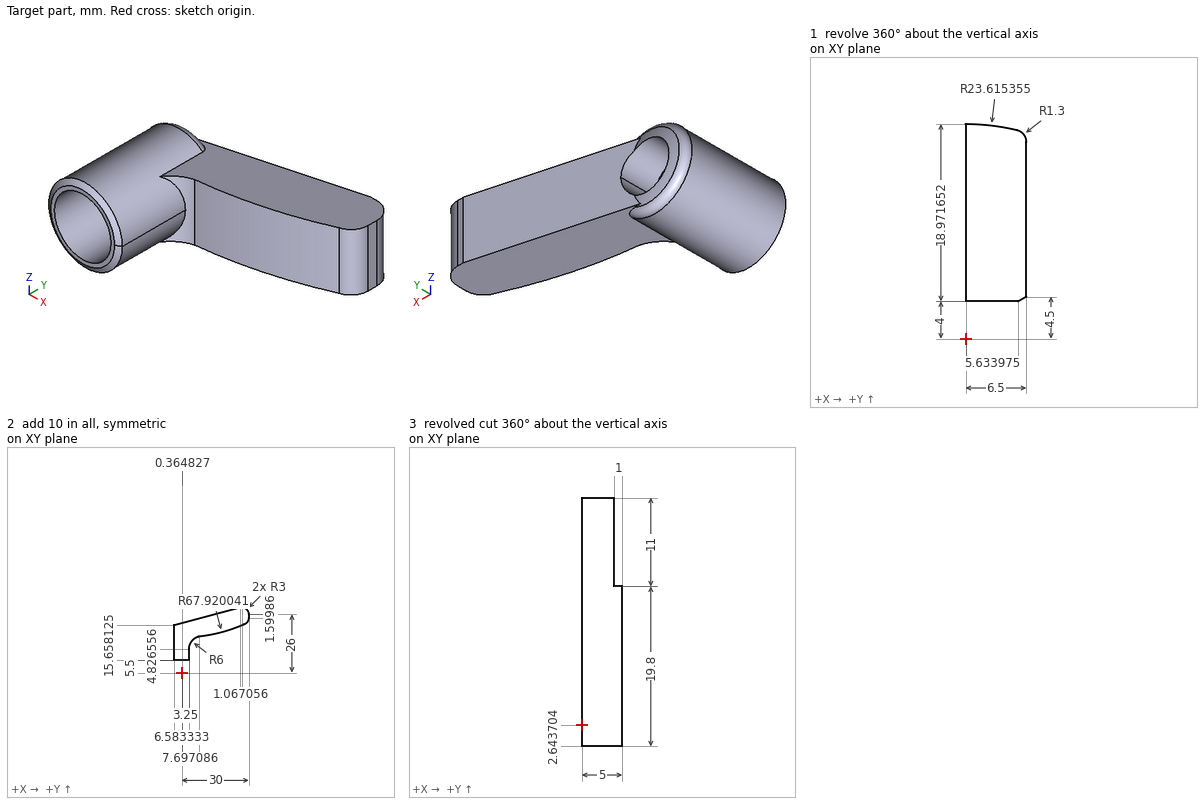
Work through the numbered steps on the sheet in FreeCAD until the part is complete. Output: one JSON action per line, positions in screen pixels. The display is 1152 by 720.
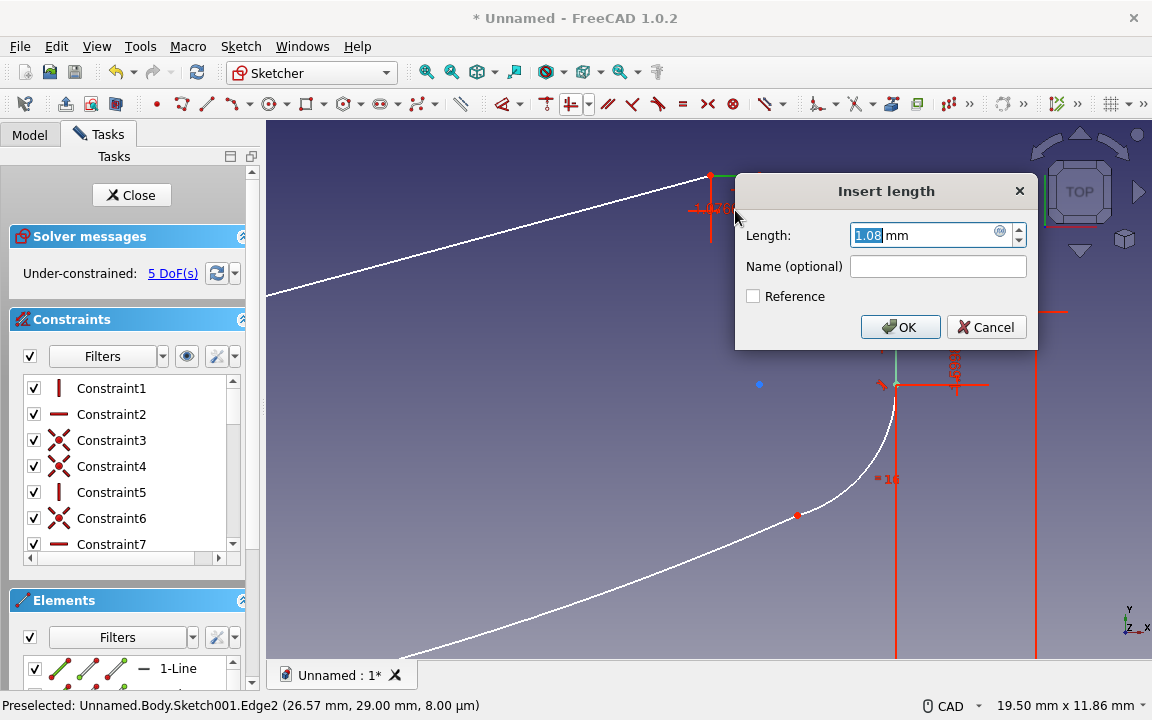
{"action": "type", "text": "1.067056"}
{"action": "key", "text": "Return"}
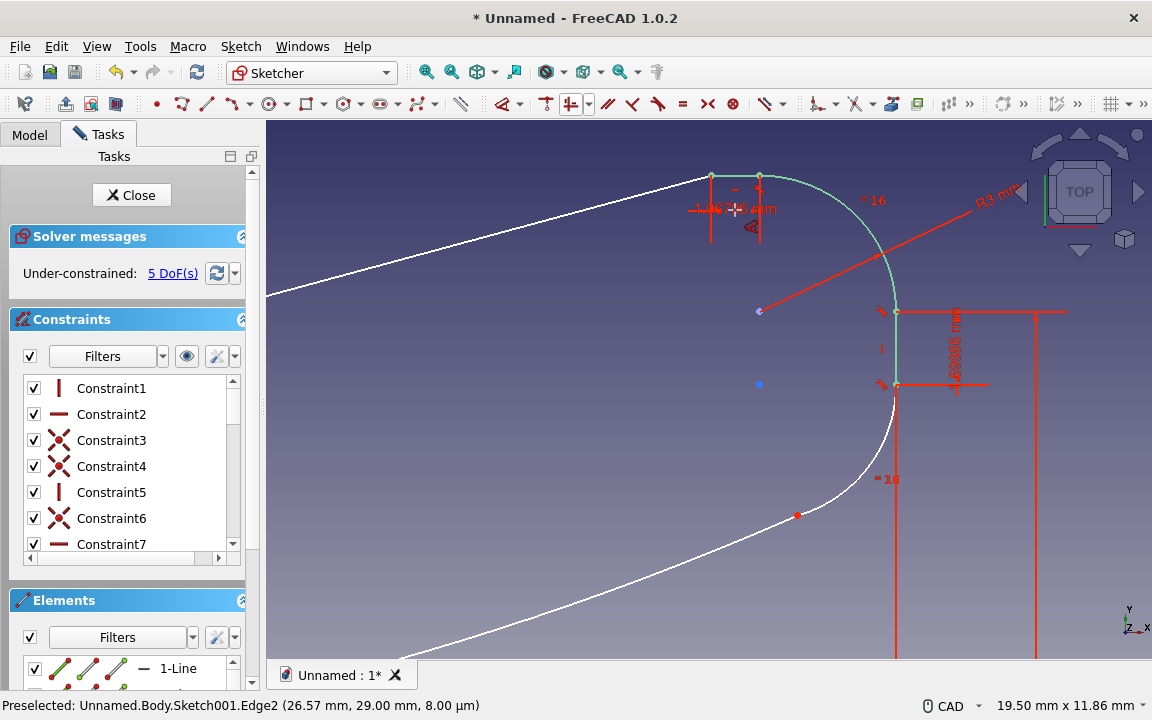
{"action": "scroll", "coordinate": [805, 244], "scroll_direction": "down", "scroll_amount": 7}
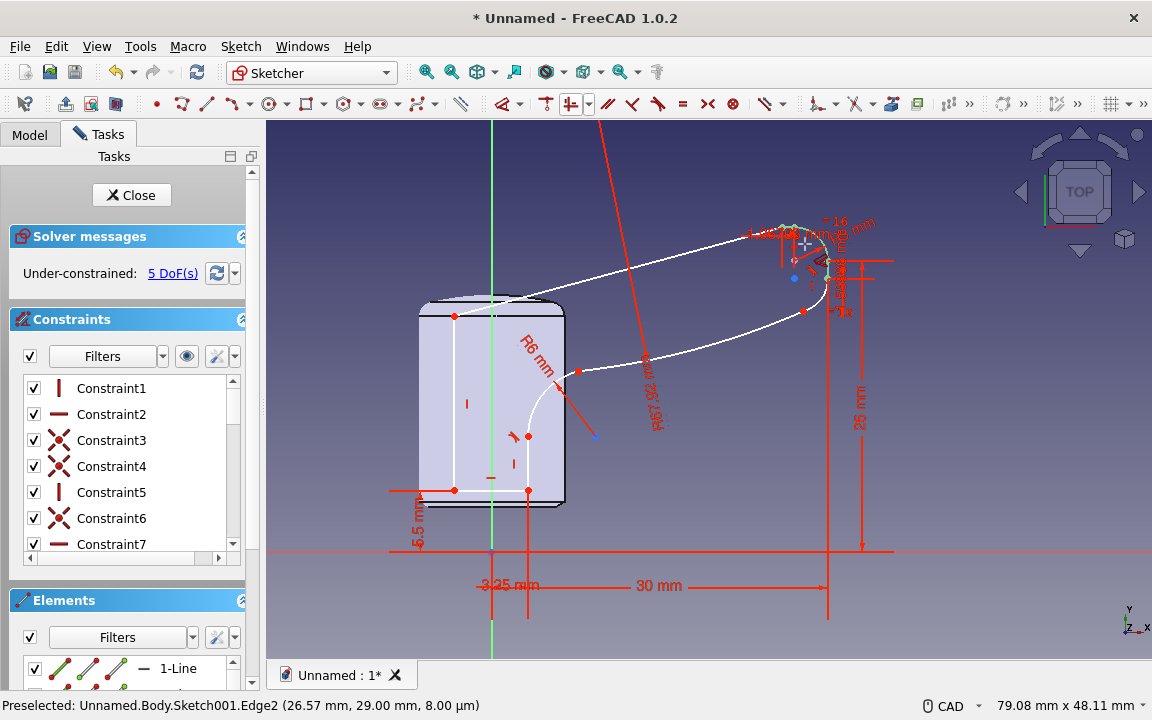
{"action": "left_click", "coordinate": [477, 491]}
{"action": "left_click", "coordinate": [508, 525]}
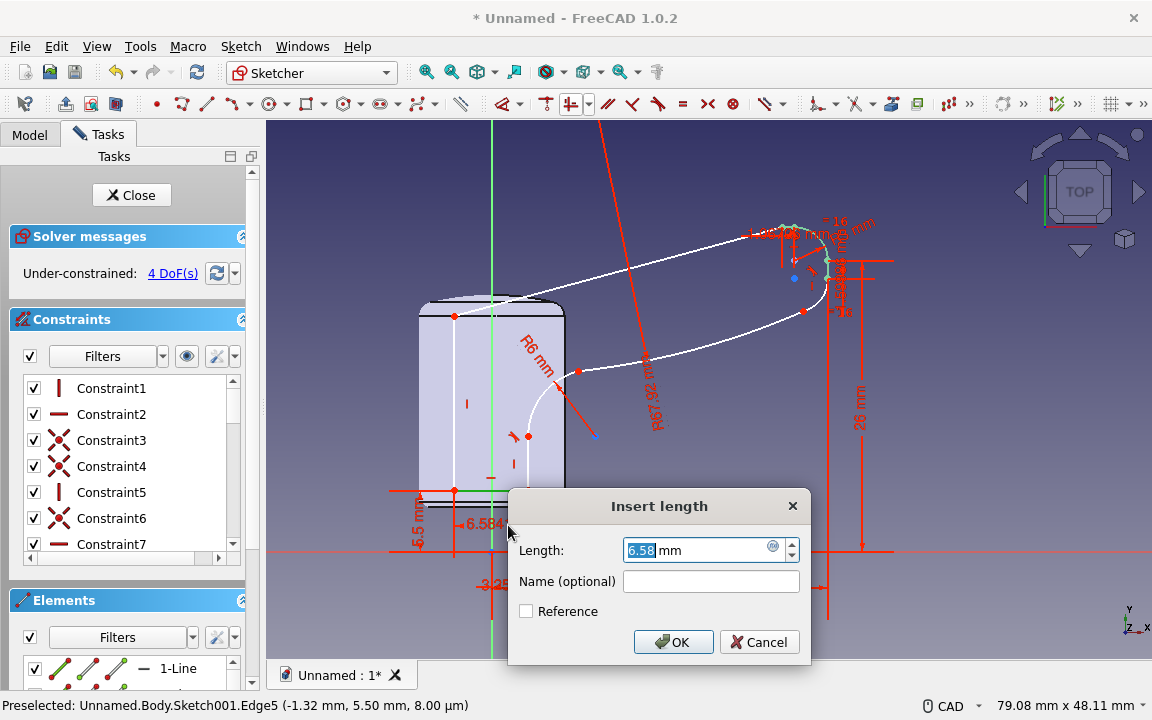
{"action": "type", "text": "6.583333"}
{"action": "key", "text": "Return"}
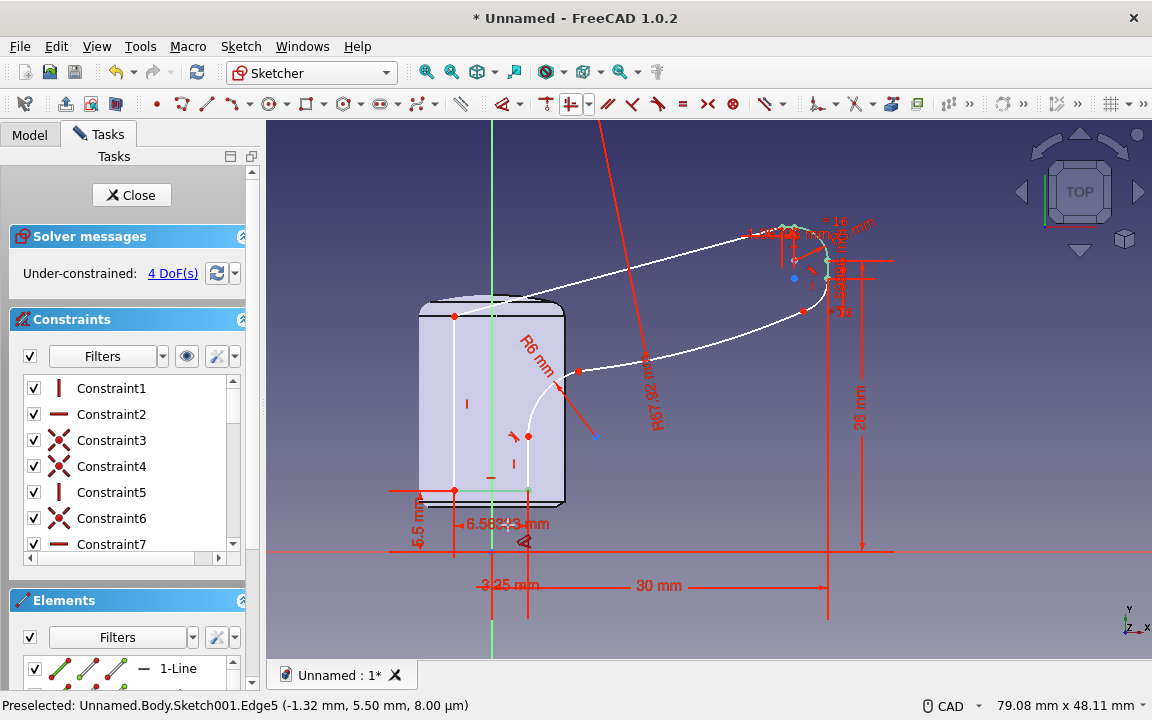
{"action": "left_click", "coordinate": [528, 474]}
{"action": "left_click", "coordinate": [562, 463]}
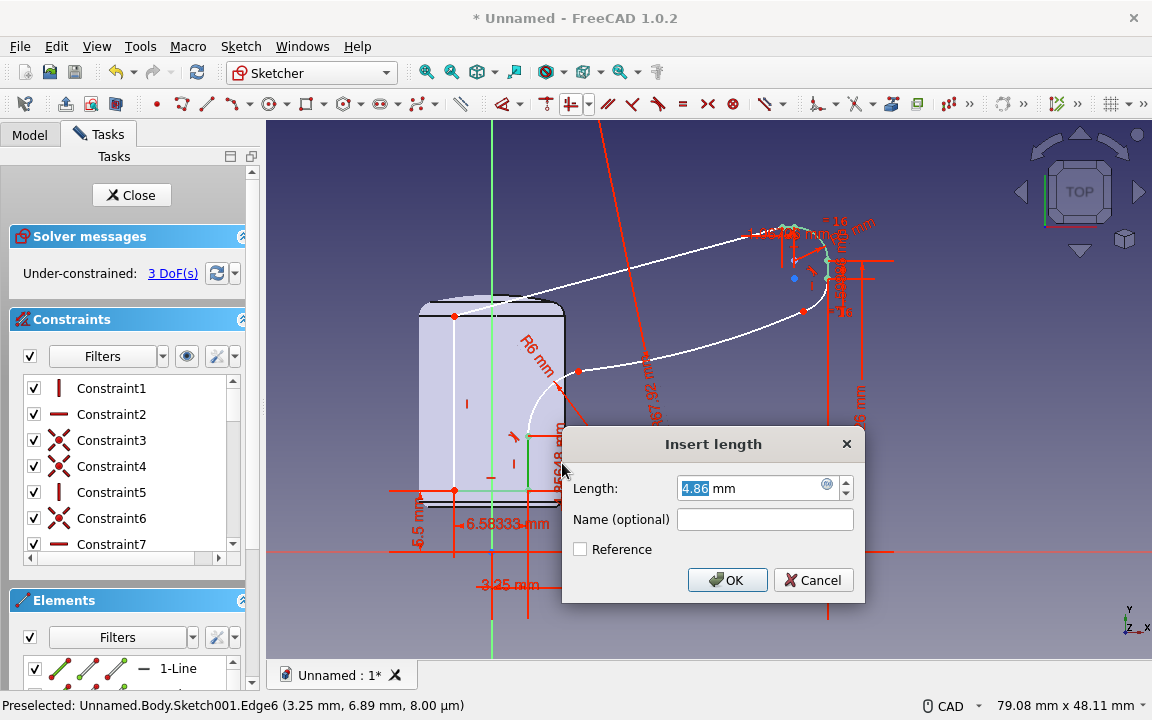
{"action": "type", "text": "4.826556"}
{"action": "key", "text": "Return"}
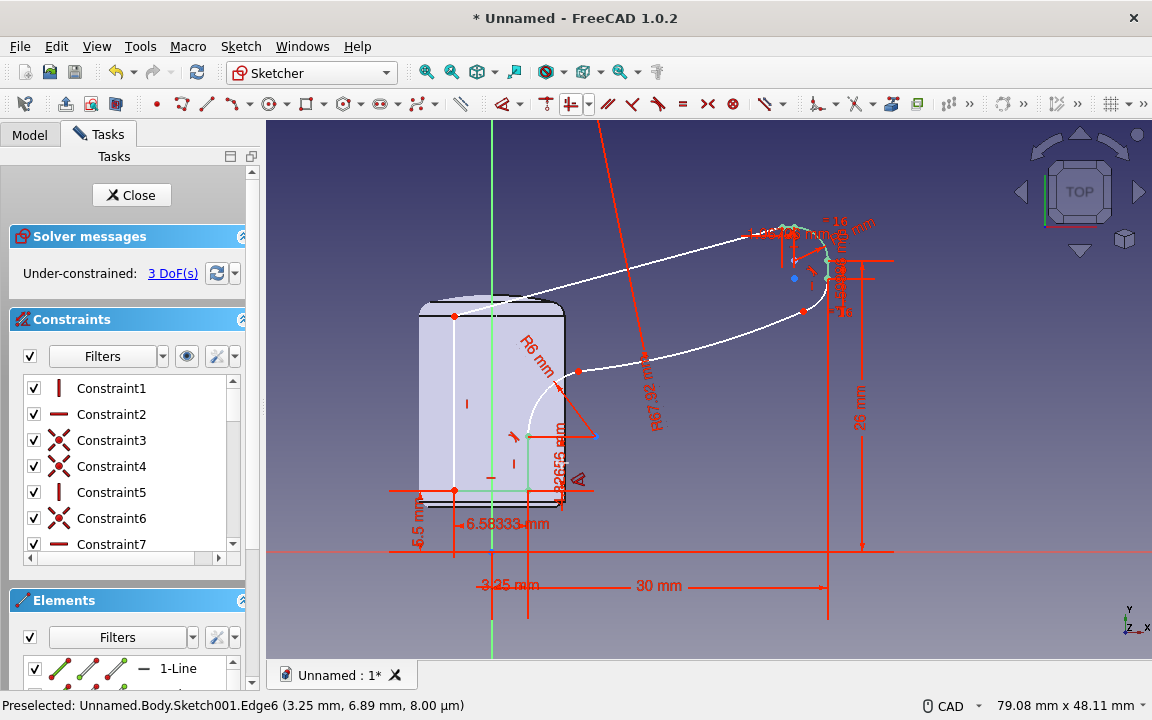
{"action": "left_click", "coordinate": [454, 368]}
{"action": "left_click", "coordinate": [420, 403]}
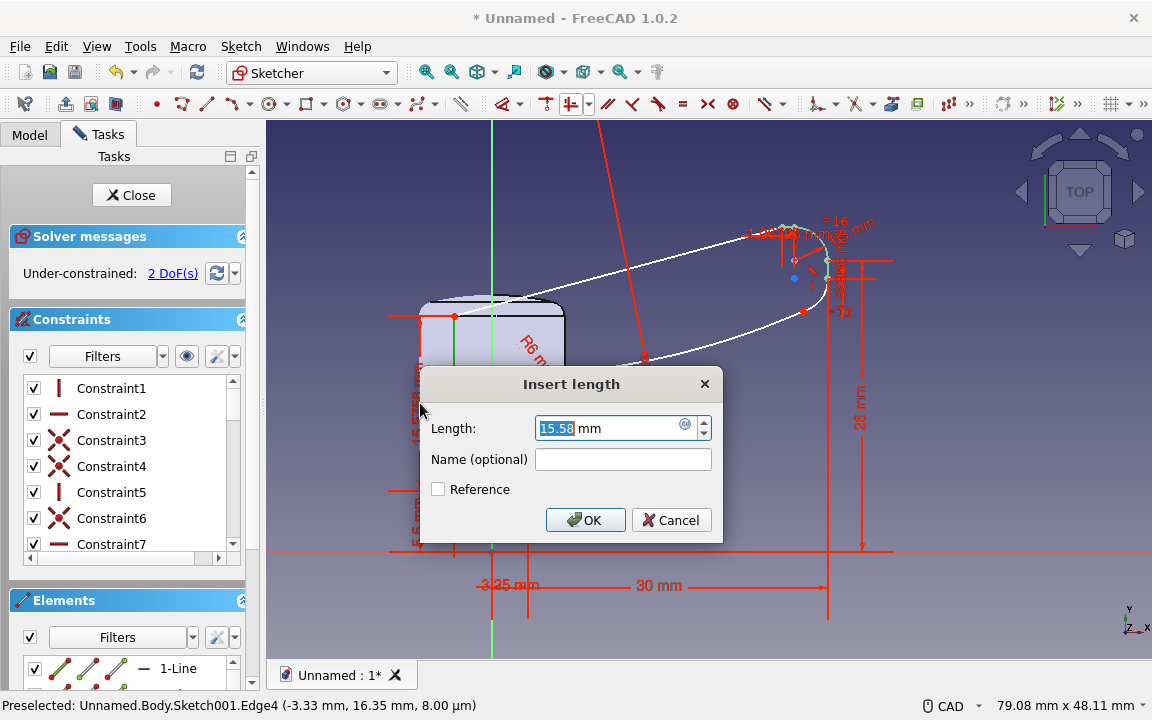
{"action": "type", "text": "15.658125"}
{"action": "key", "text": "Return"}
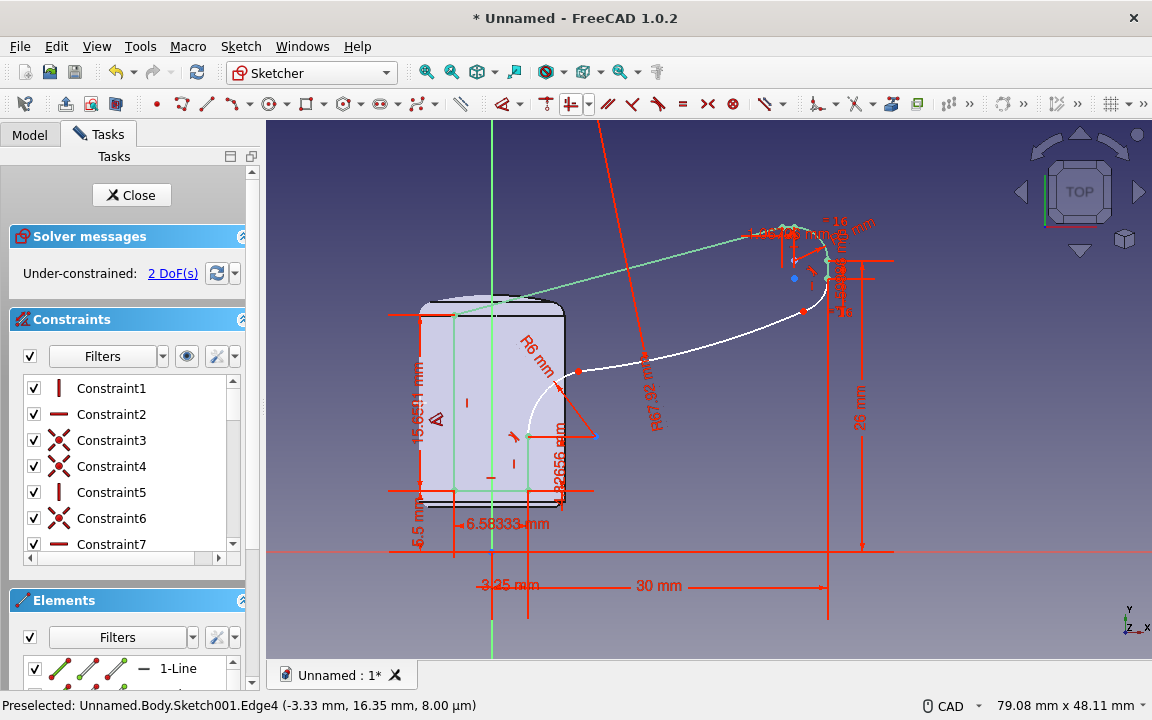
{"action": "left_click", "coordinate": [578, 372]}
{"action": "left_click", "coordinate": [535, 610]}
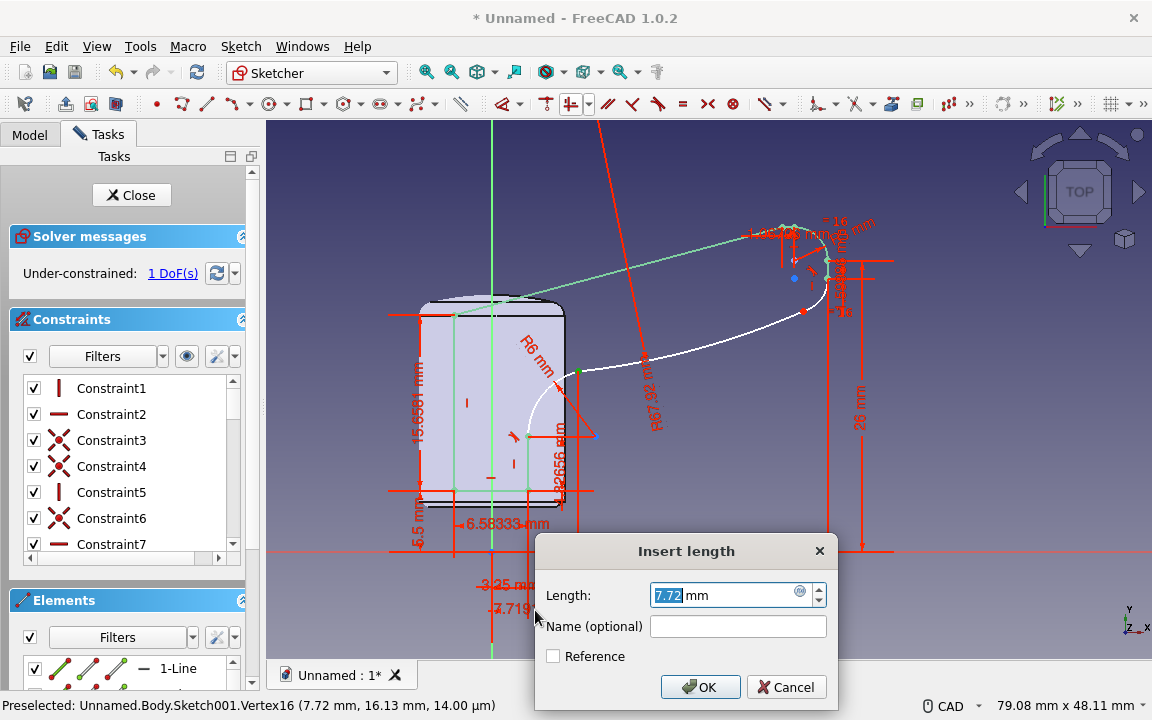
{"action": "type", "text": "7.697086"}
{"action": "key", "text": "Return"}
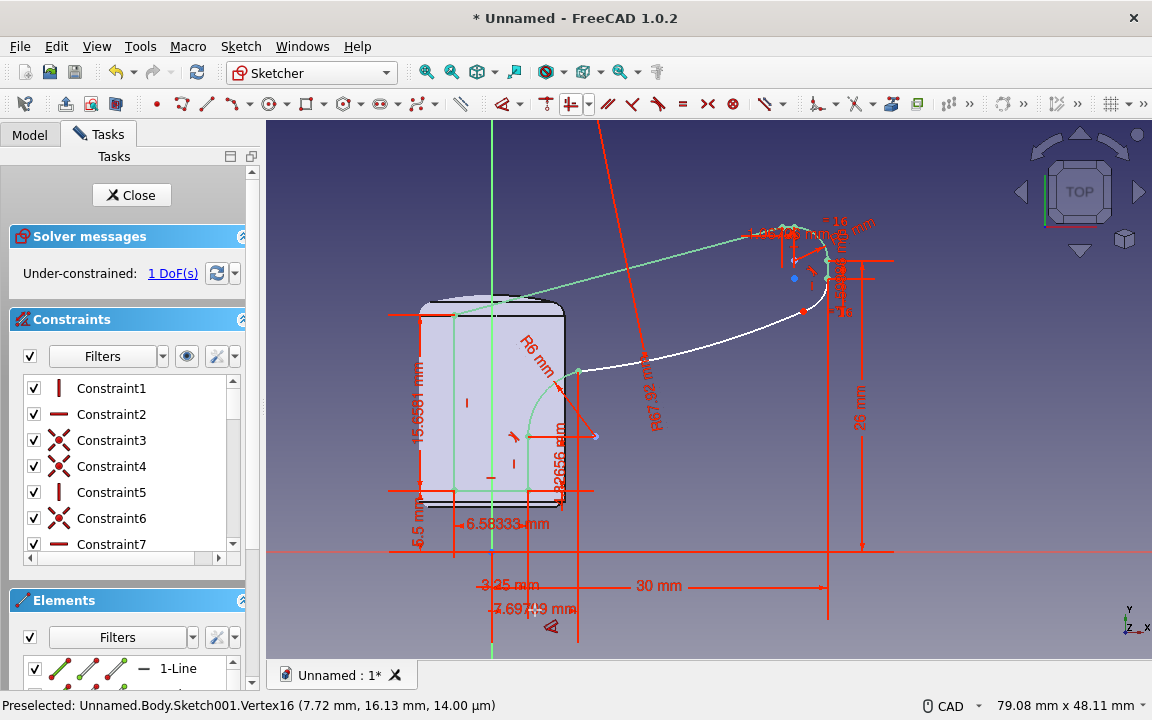
{"action": "scroll", "coordinate": [640, 567], "scroll_direction": "down", "scroll_amount": 5}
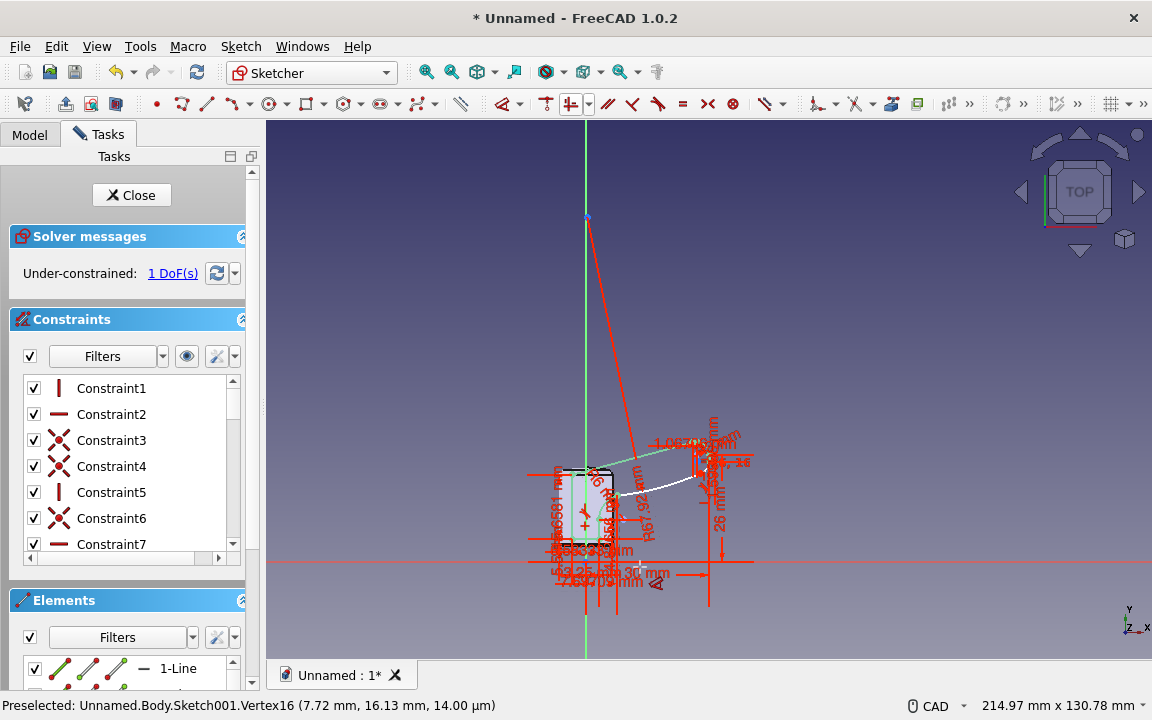
{"action": "scroll", "coordinate": [587, 217], "scroll_direction": "up", "scroll_amount": 17}